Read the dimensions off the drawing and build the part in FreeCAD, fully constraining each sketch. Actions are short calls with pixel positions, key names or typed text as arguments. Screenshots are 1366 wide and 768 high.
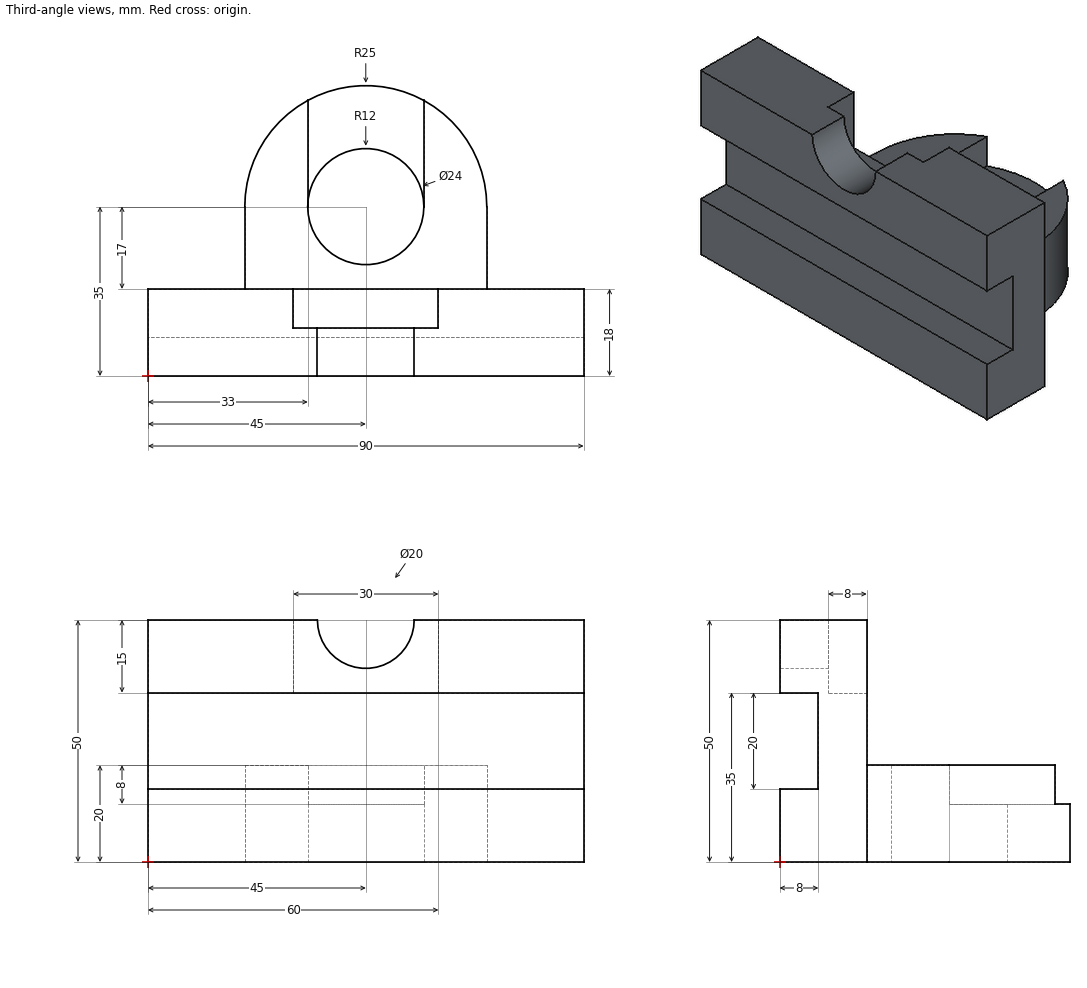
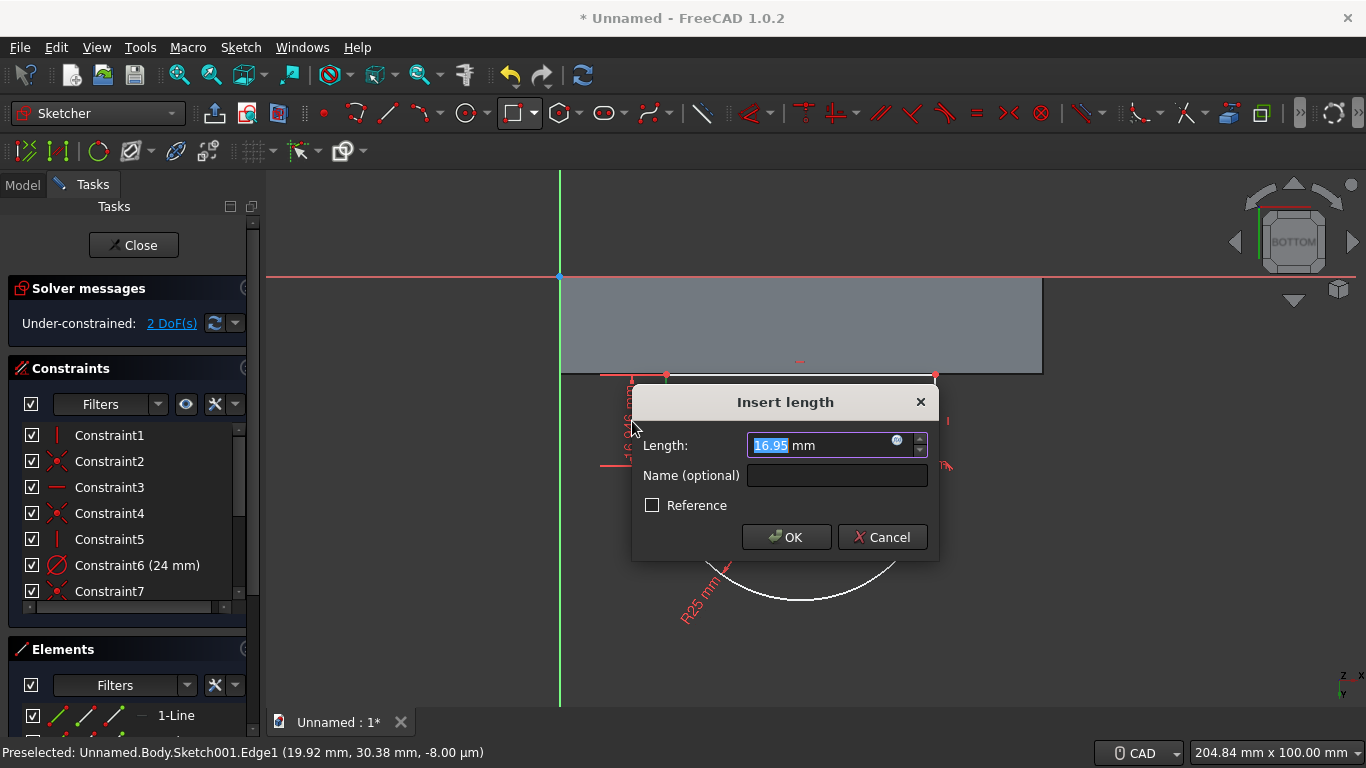
text(17)
key(Return)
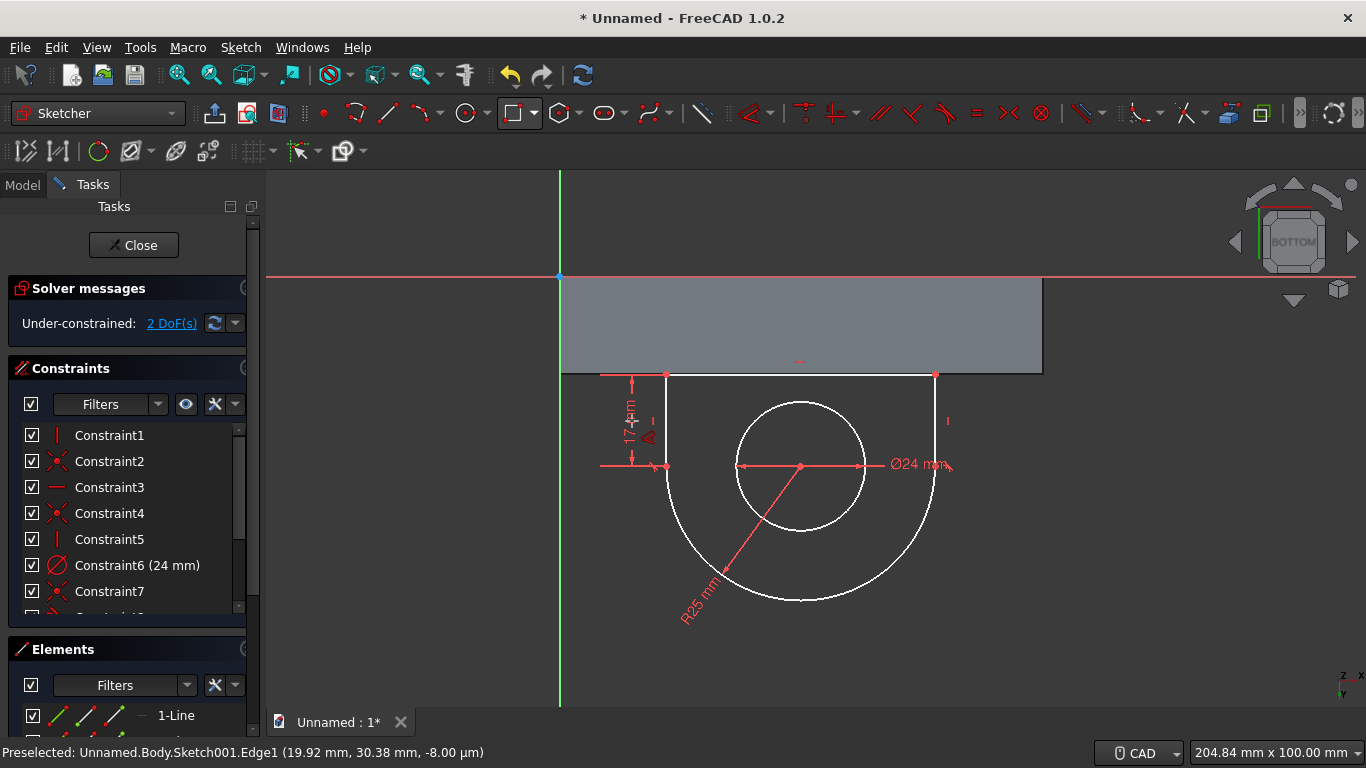
click(801, 466)
click(680, 243)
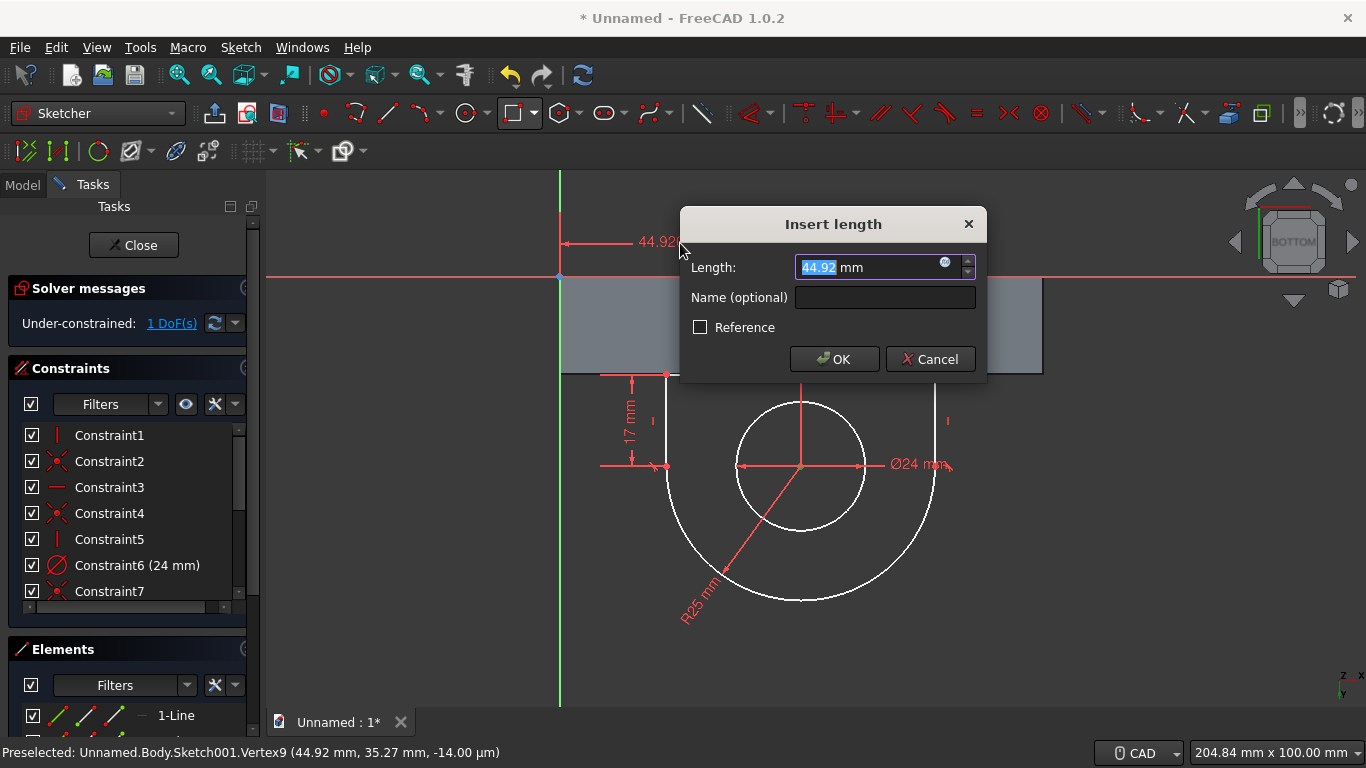
text(45)
key(Return)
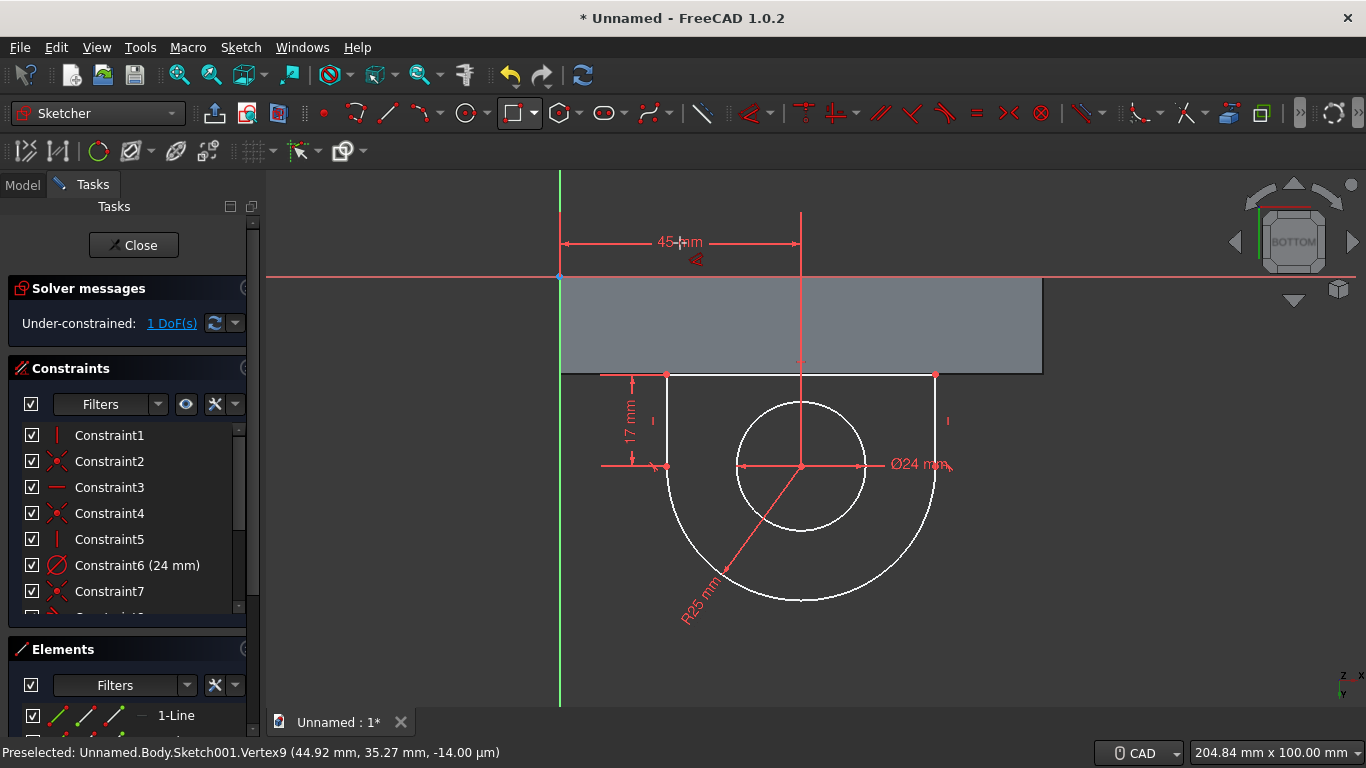
click(801, 466)
click(526, 372)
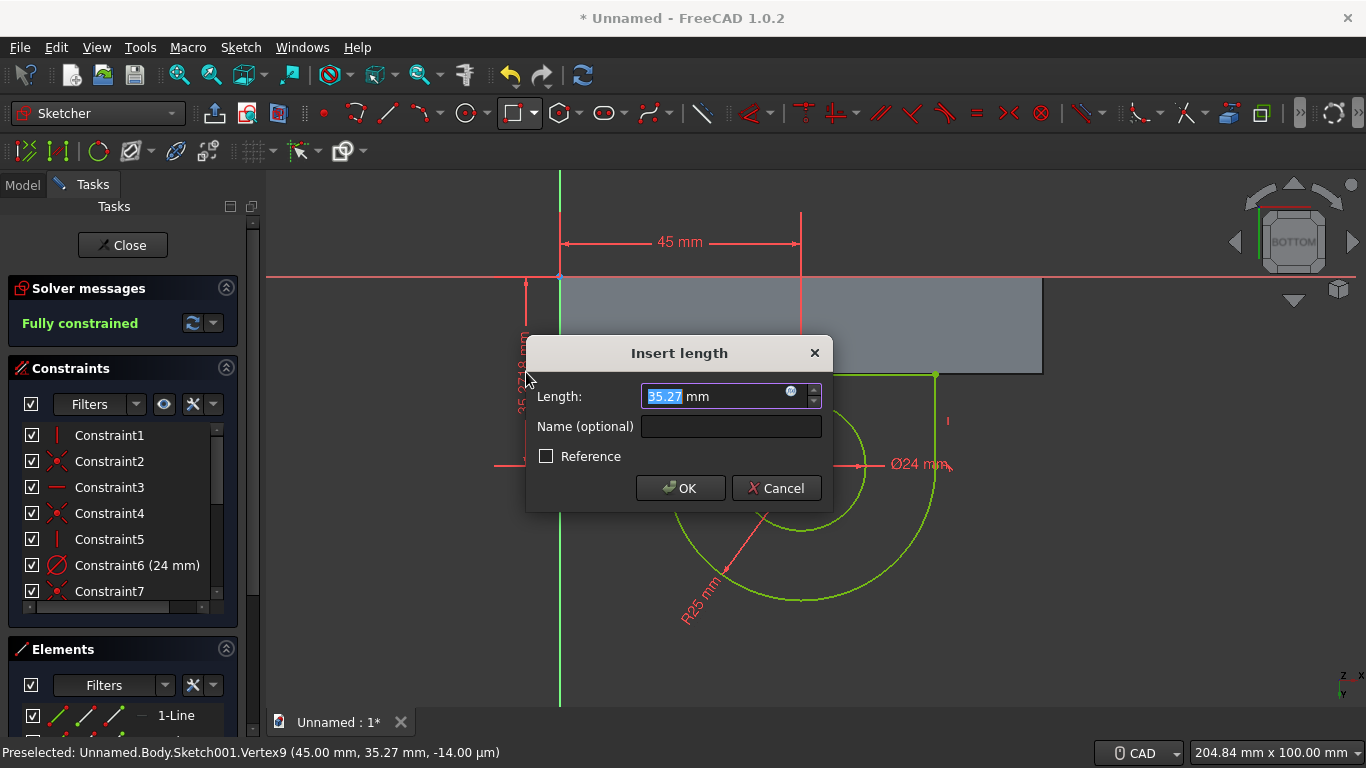
text(35)
key(Return)
key(Escape)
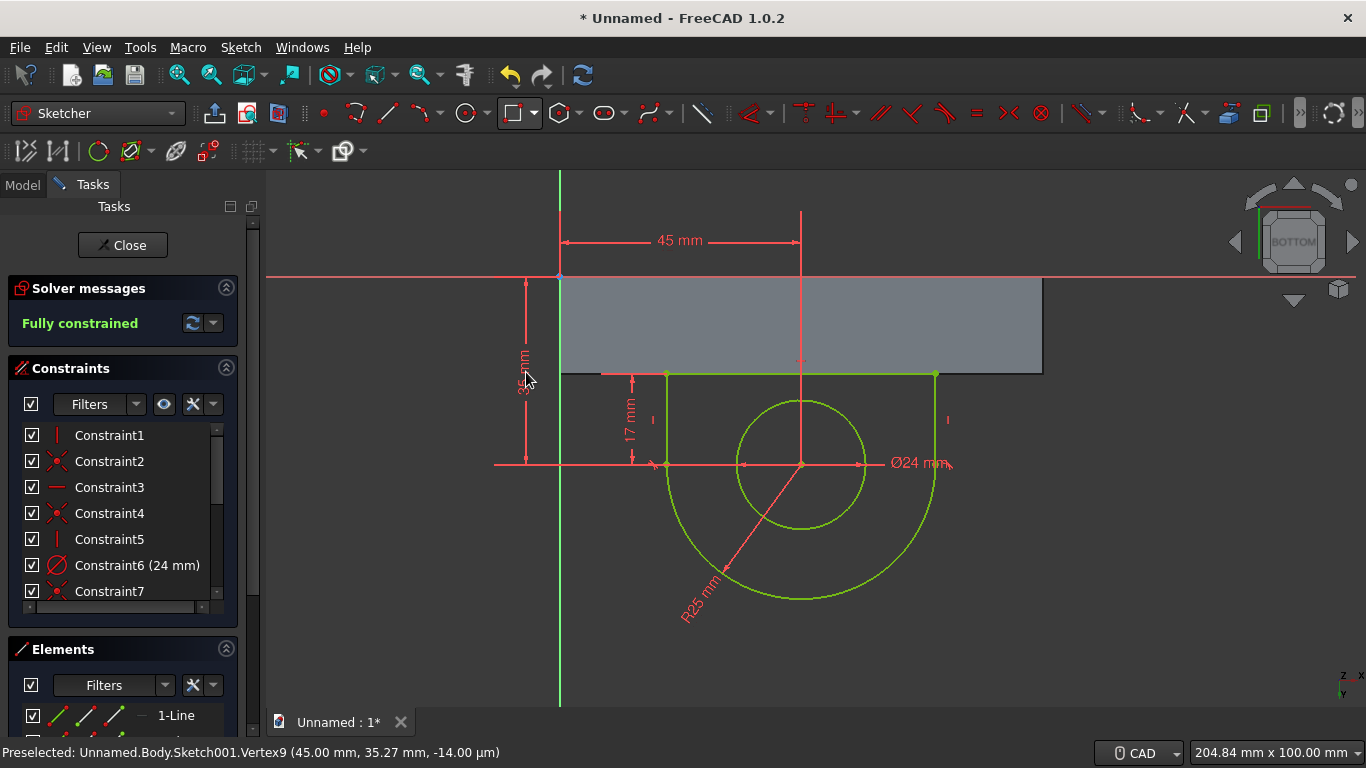
click(123, 245)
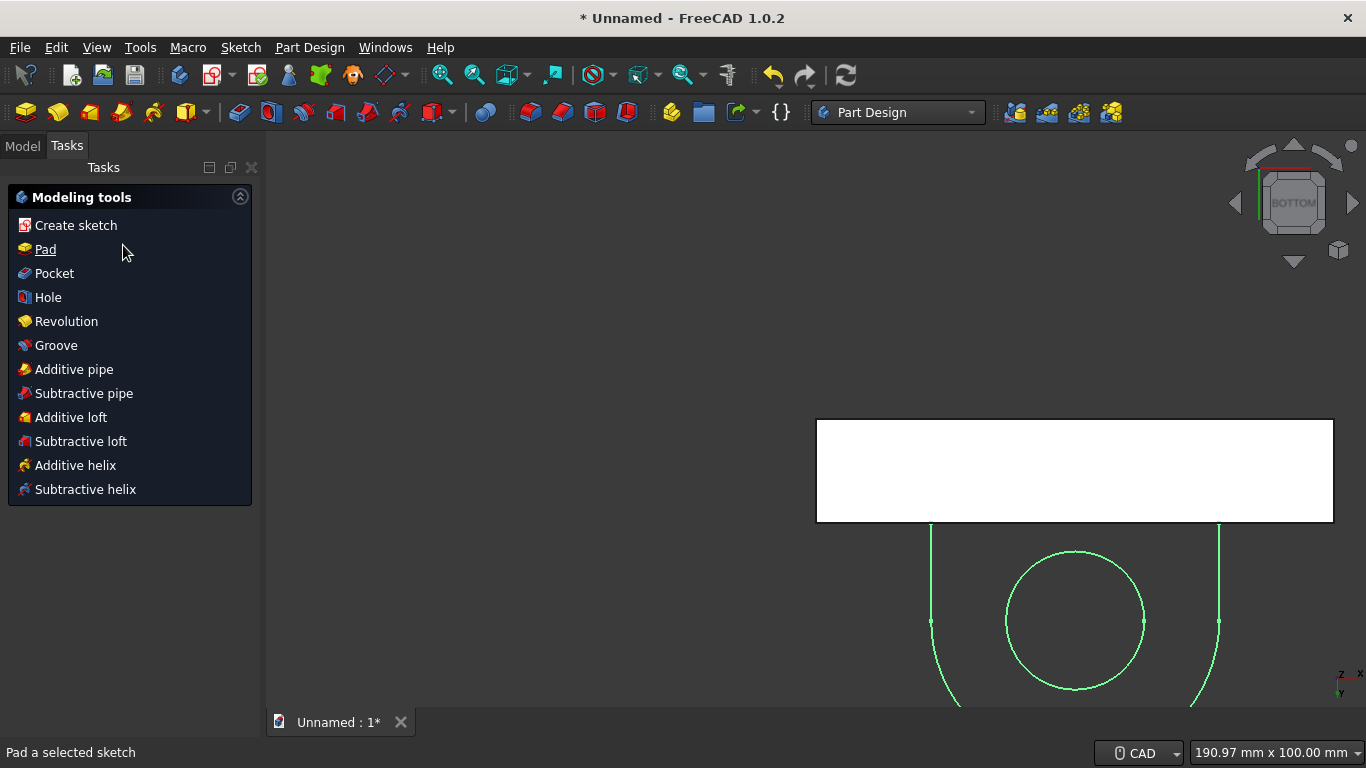
click(26, 112)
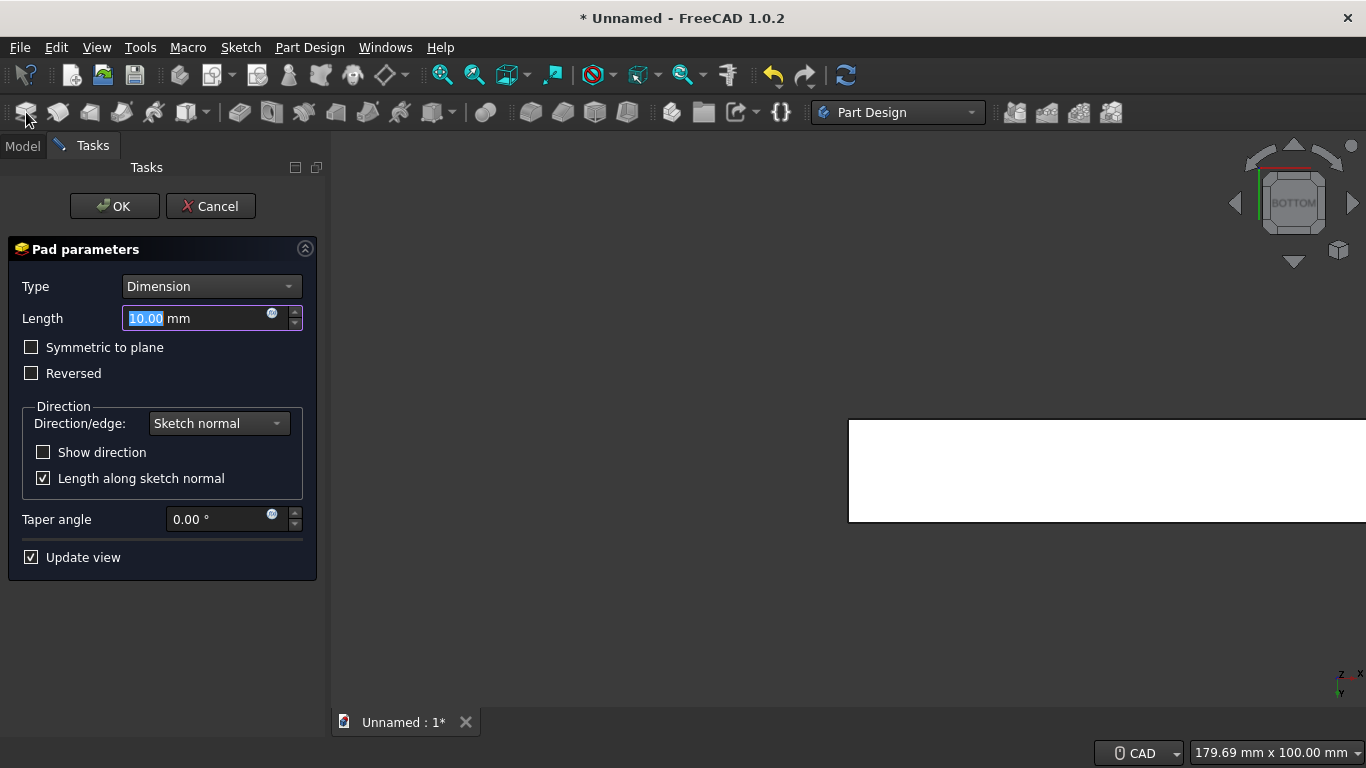
text(20)
key(Tab)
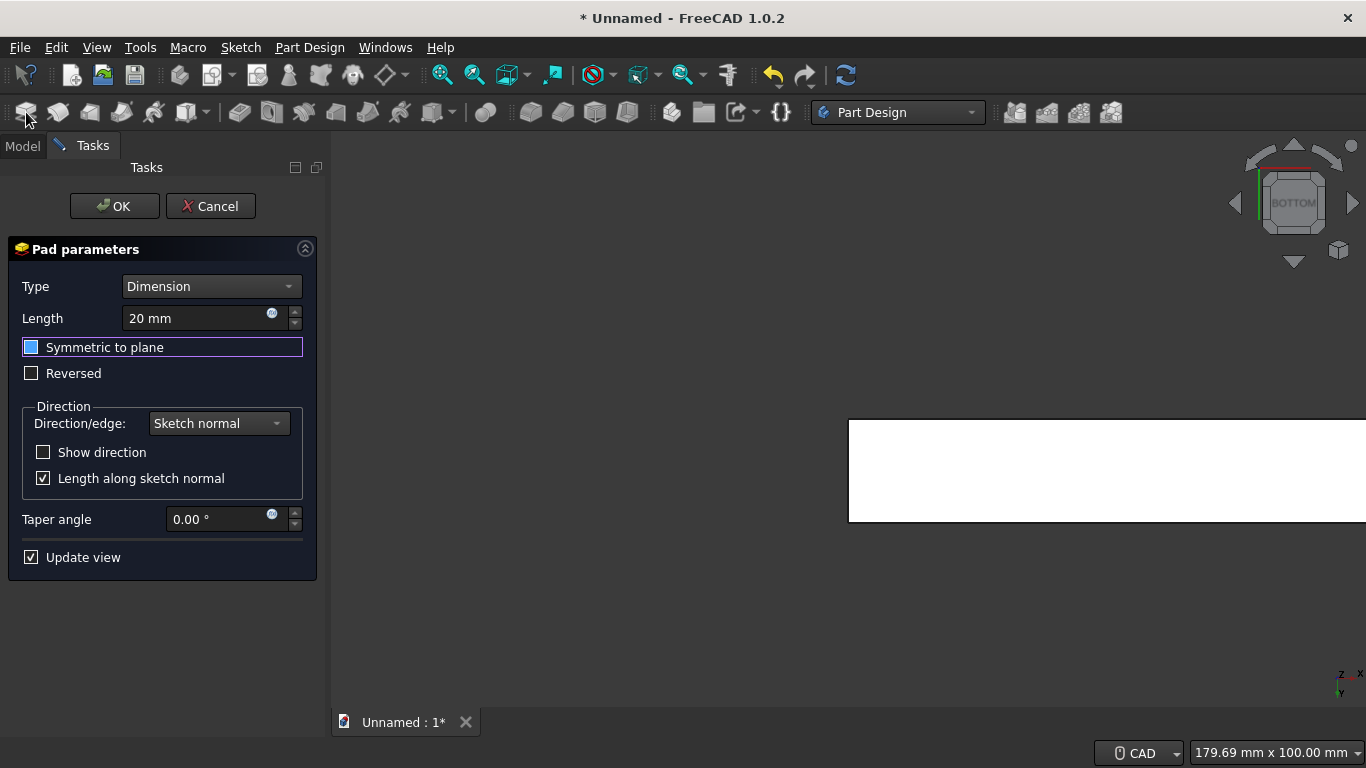
click(30, 373)